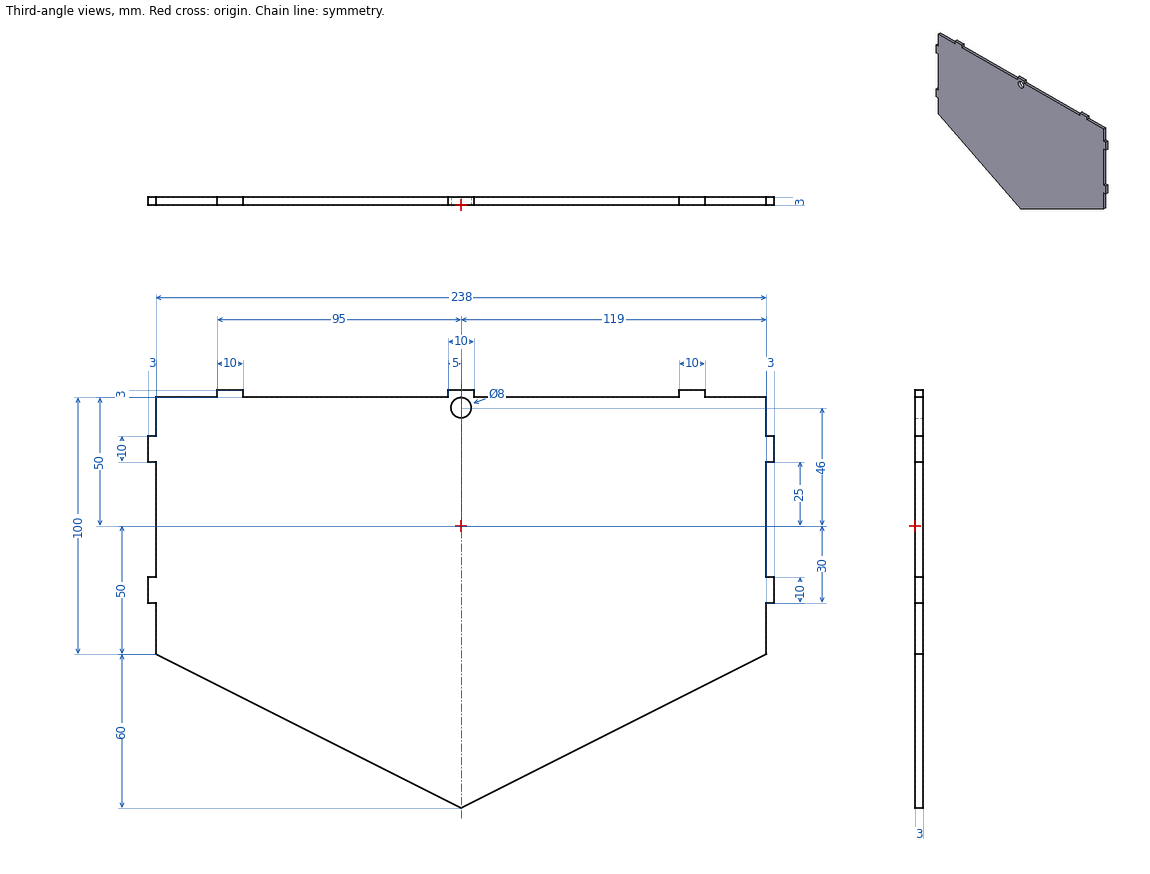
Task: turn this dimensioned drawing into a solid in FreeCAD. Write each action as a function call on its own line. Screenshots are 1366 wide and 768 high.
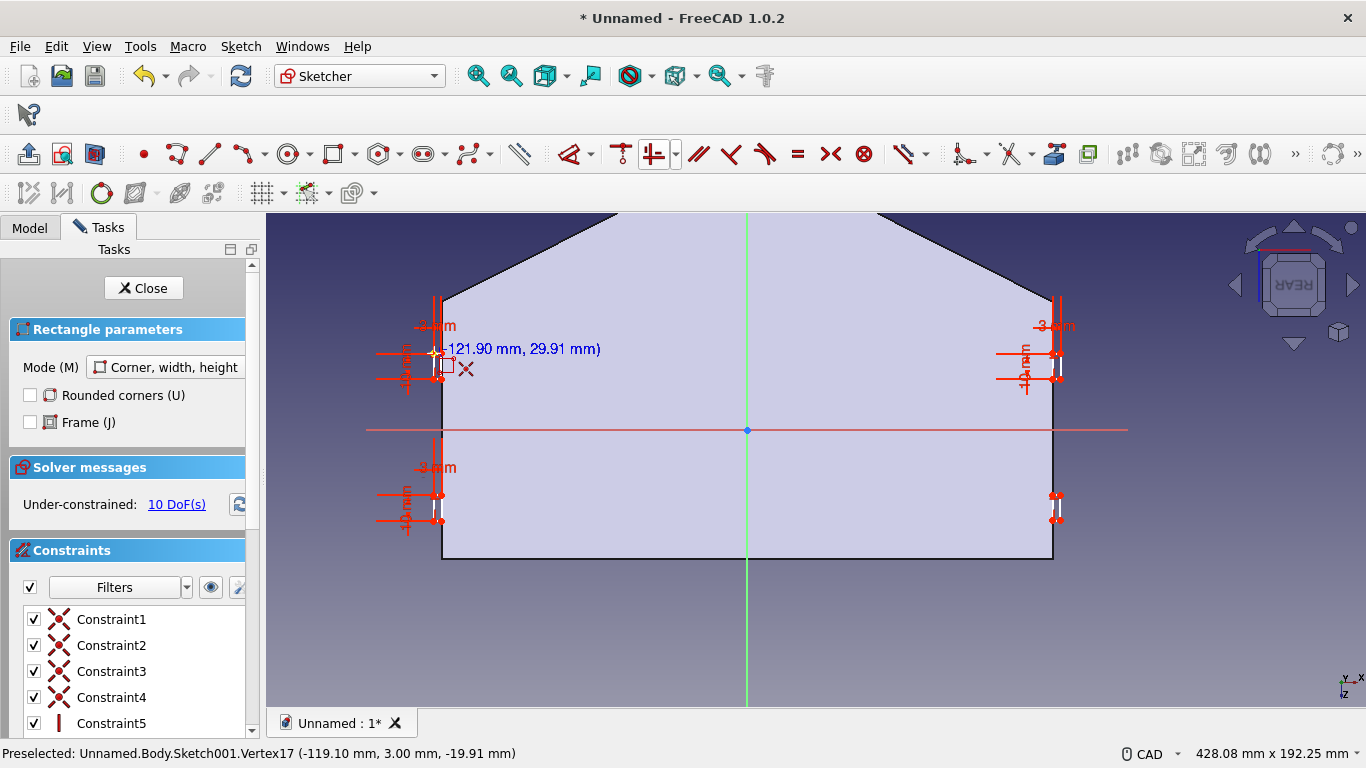
scroll(503, 559, up, 4)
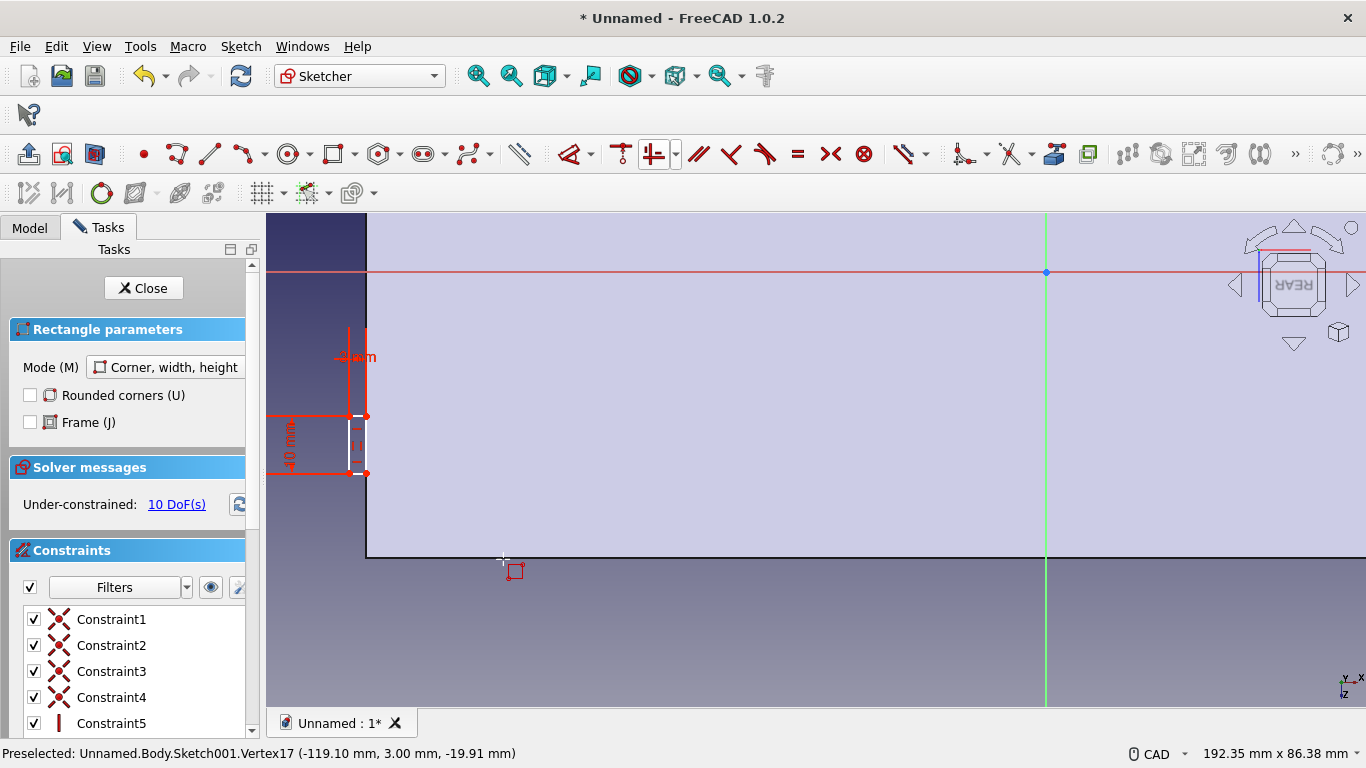
click(503, 558)
move(560, 575)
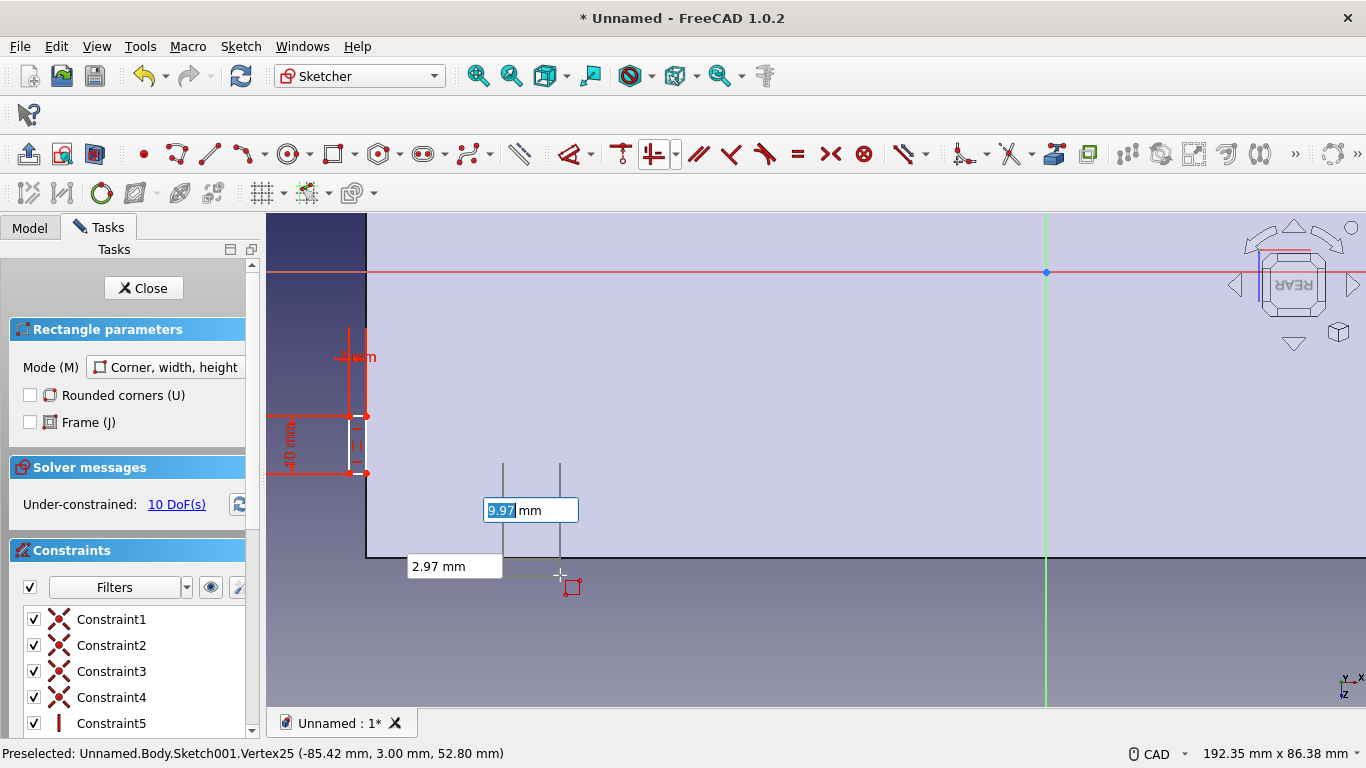
text(10)
key(Tab)
text(3)
key(Return)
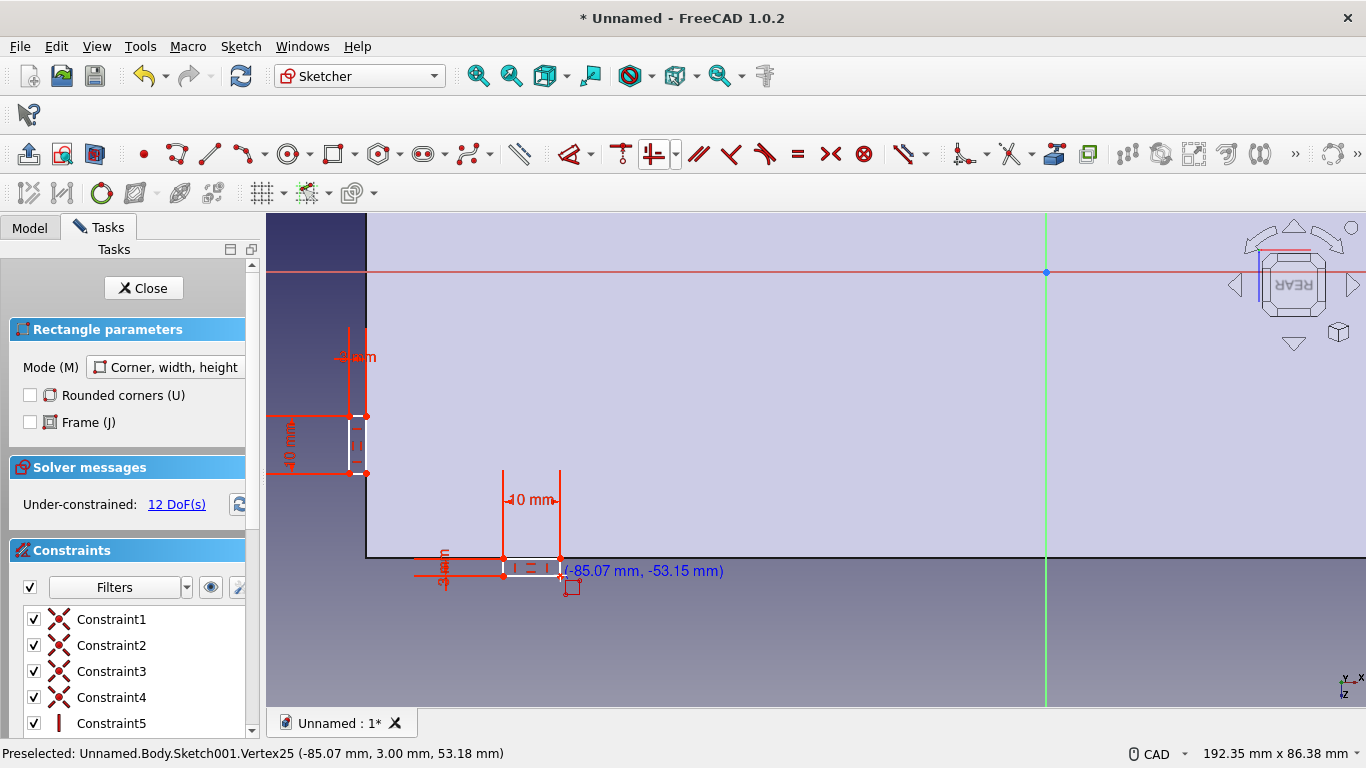
scroll(504, 560, down, 4)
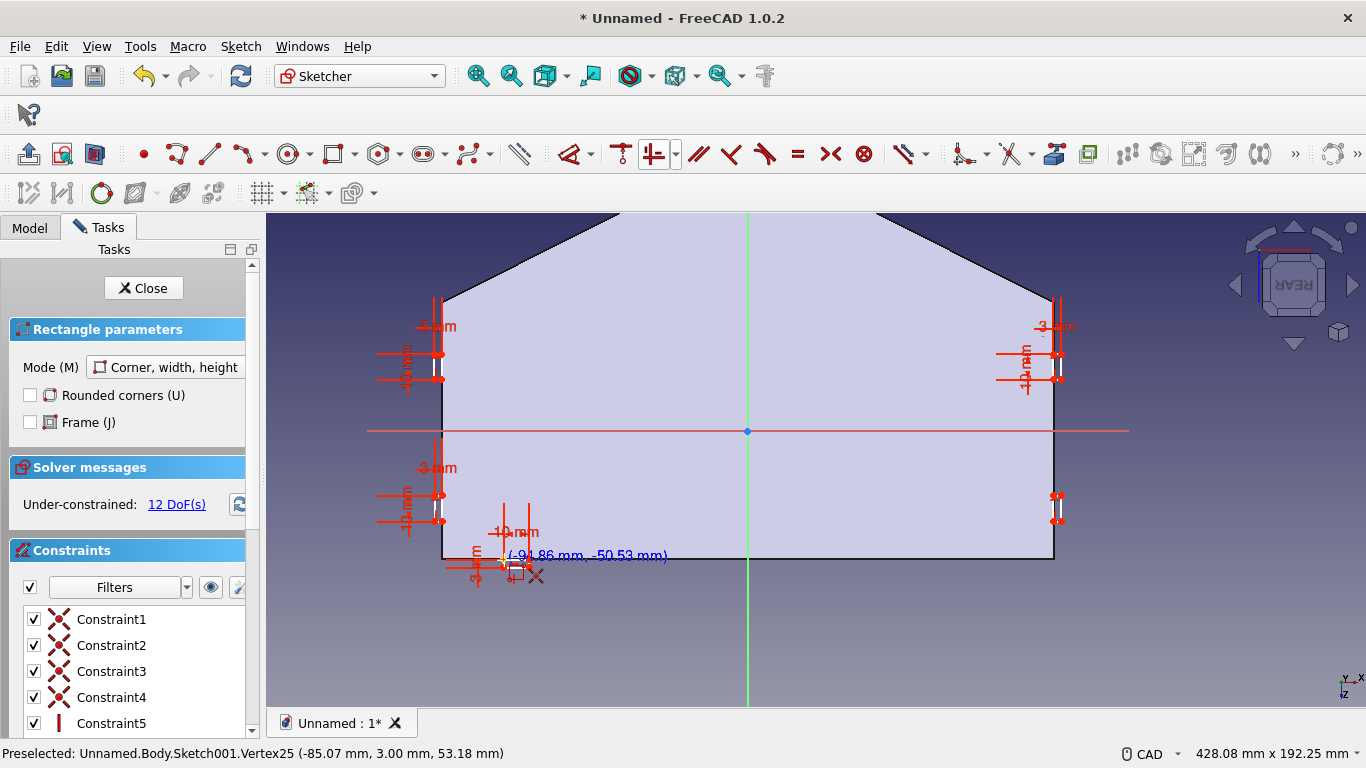
scroll(966, 559, up, 4)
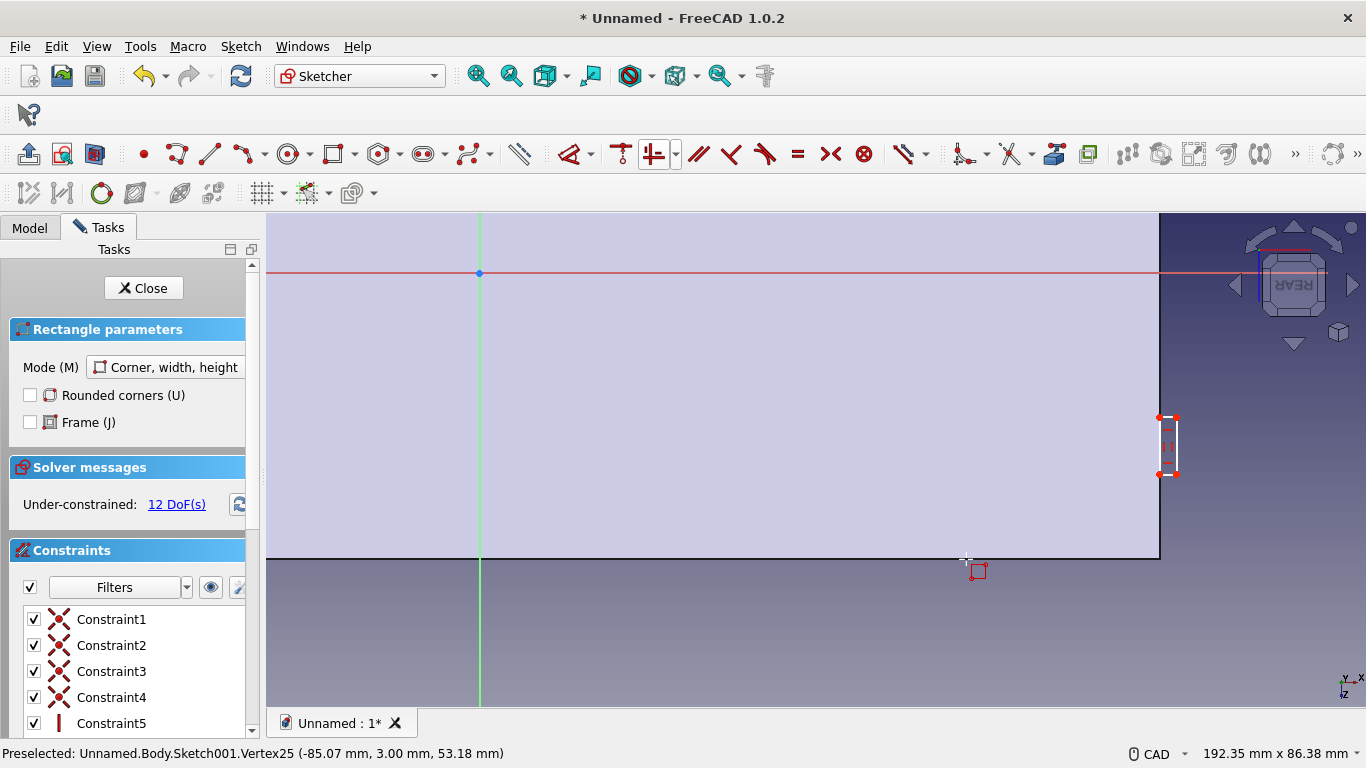
click(966, 559)
move(1023, 576)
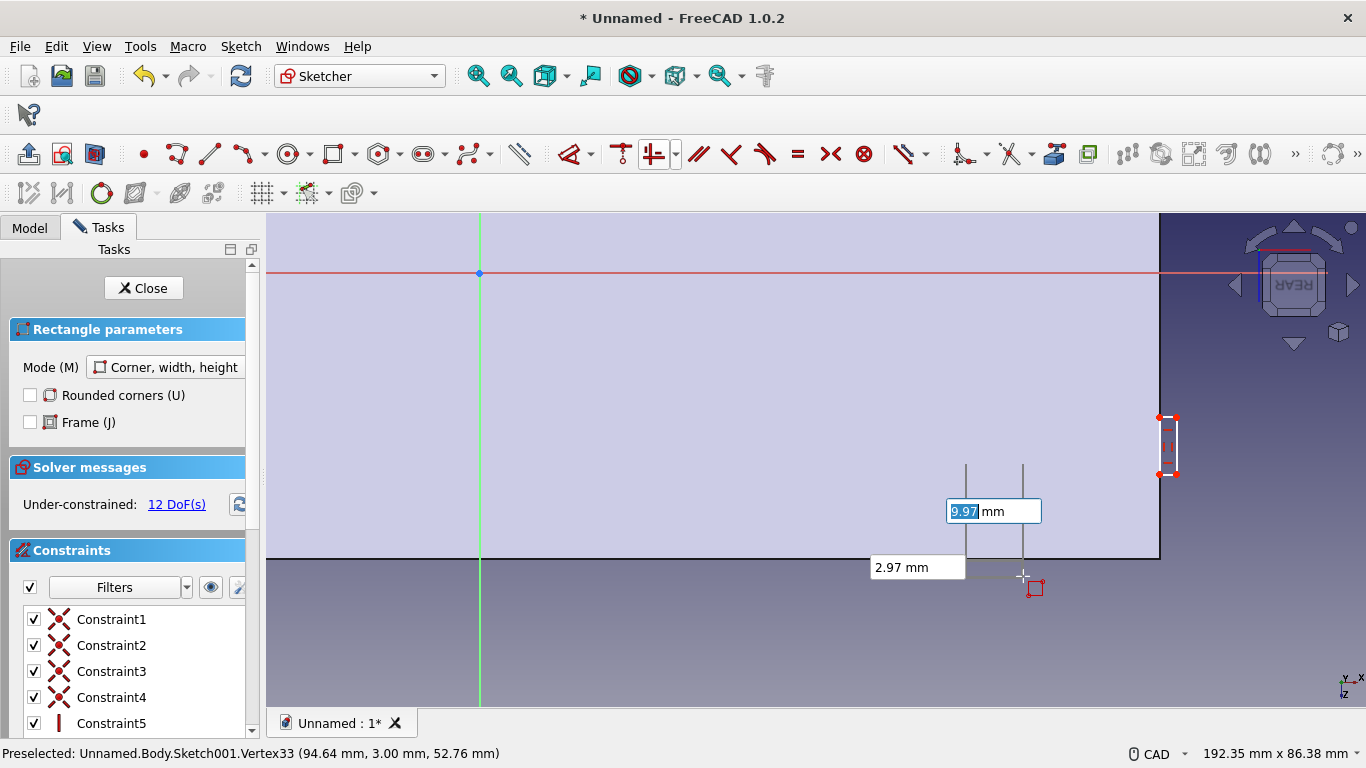
text(10)
key(Tab)
text(3)
key(Return)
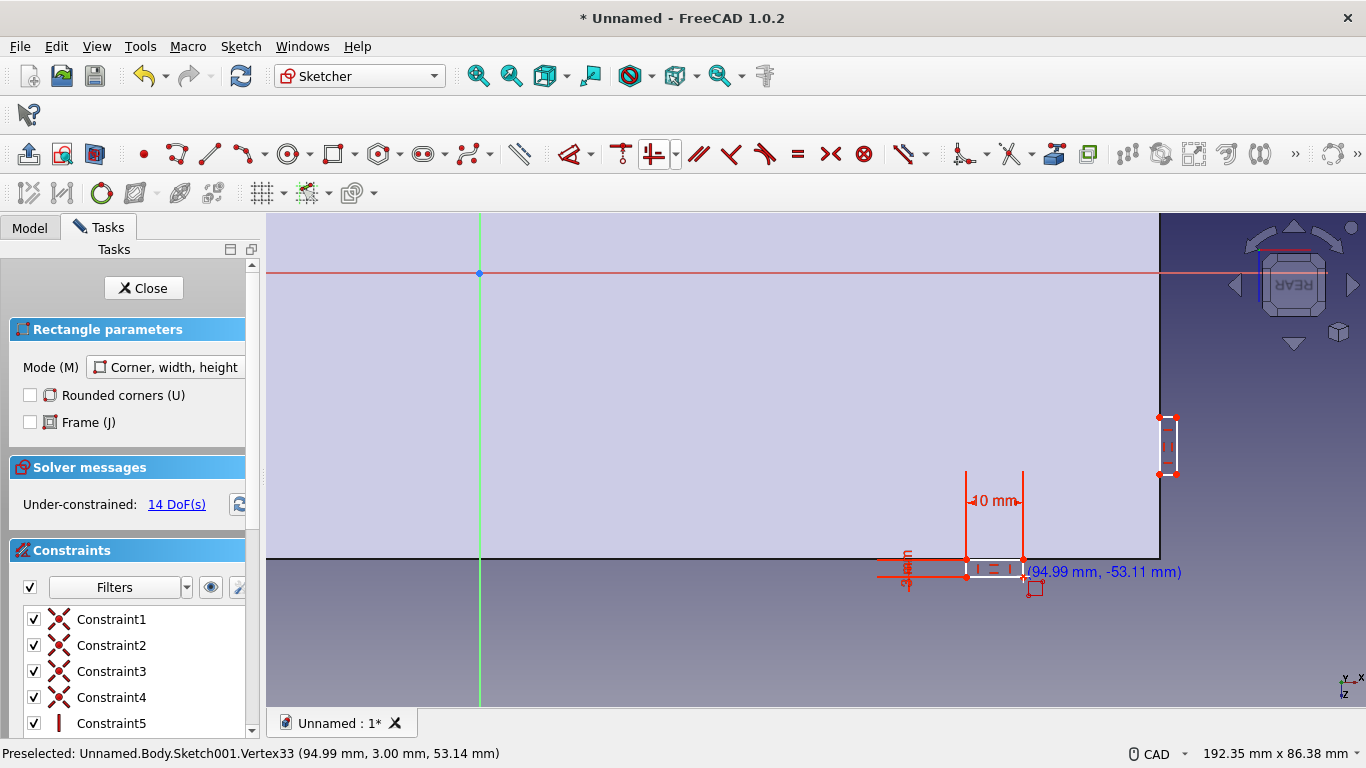
click(451, 559)
move(508, 576)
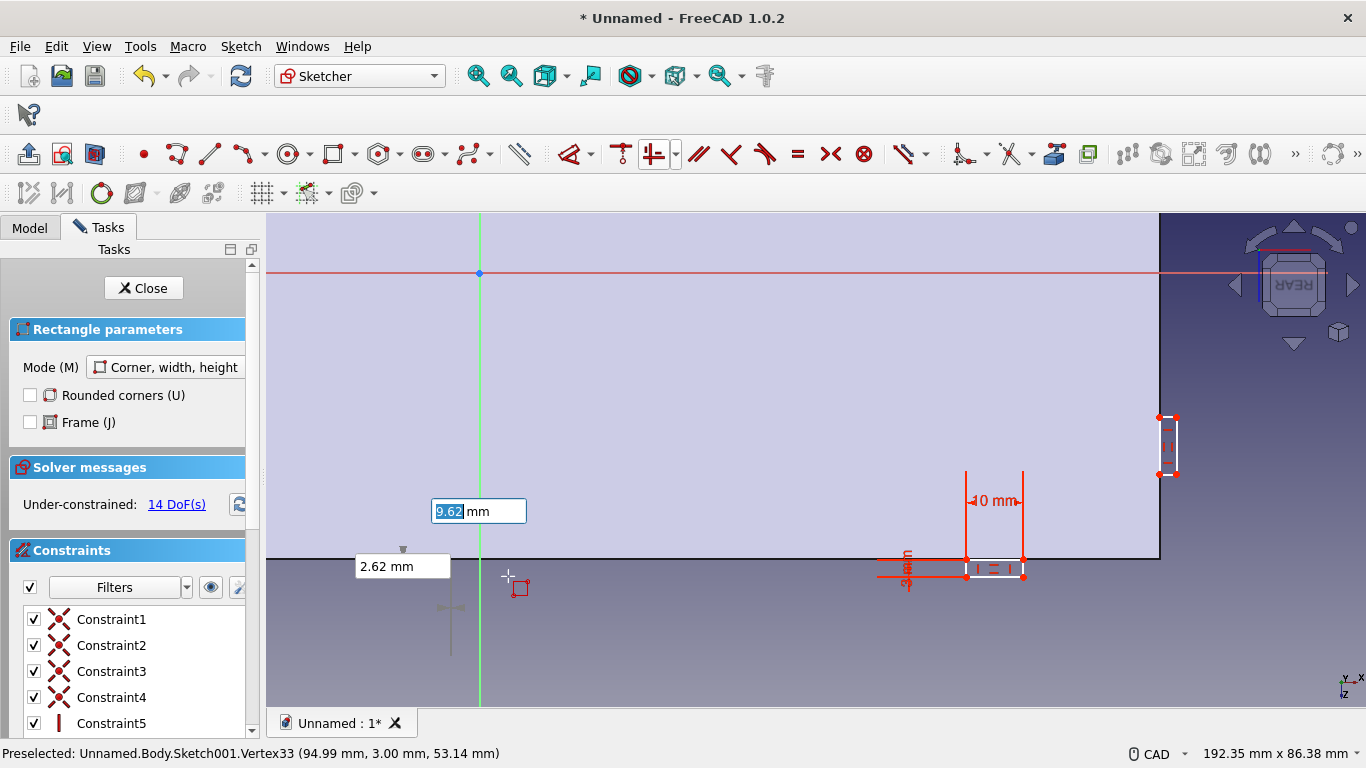
text(10)
key(Tab)
text(3)
key(Return)
key(Escape)